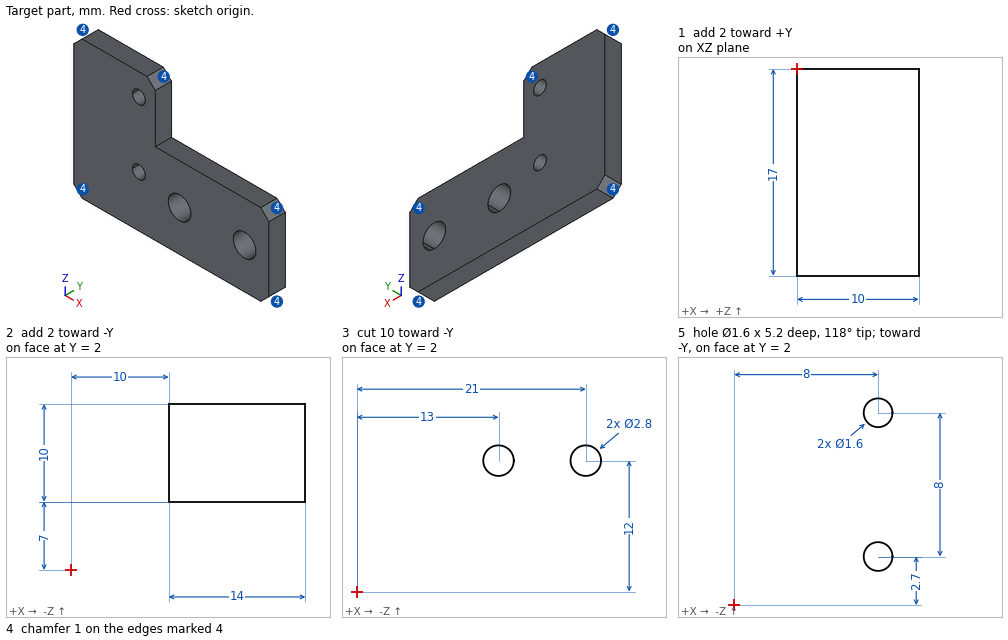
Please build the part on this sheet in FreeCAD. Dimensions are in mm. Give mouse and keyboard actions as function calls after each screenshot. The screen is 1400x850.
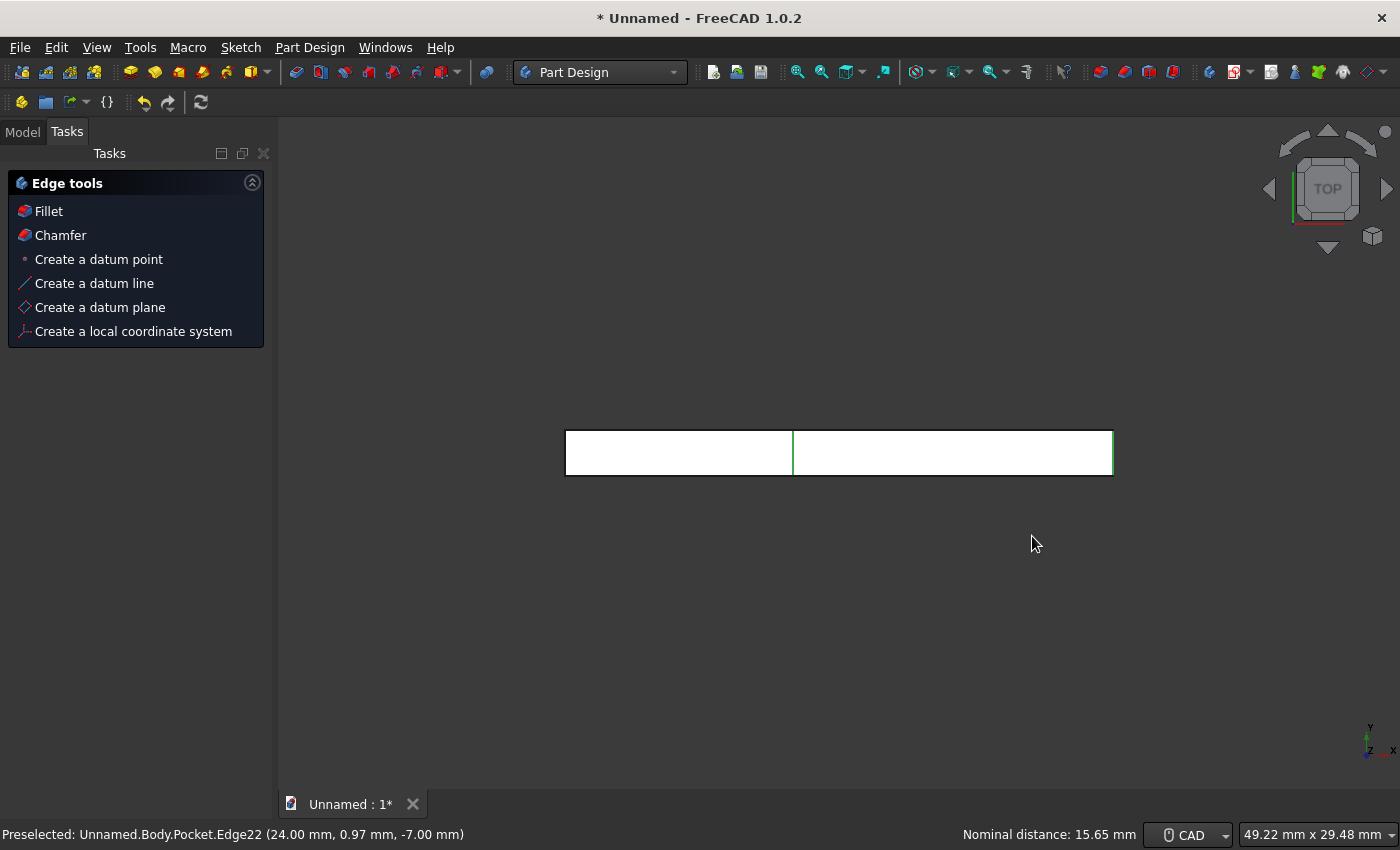
click(565, 452, ctrl)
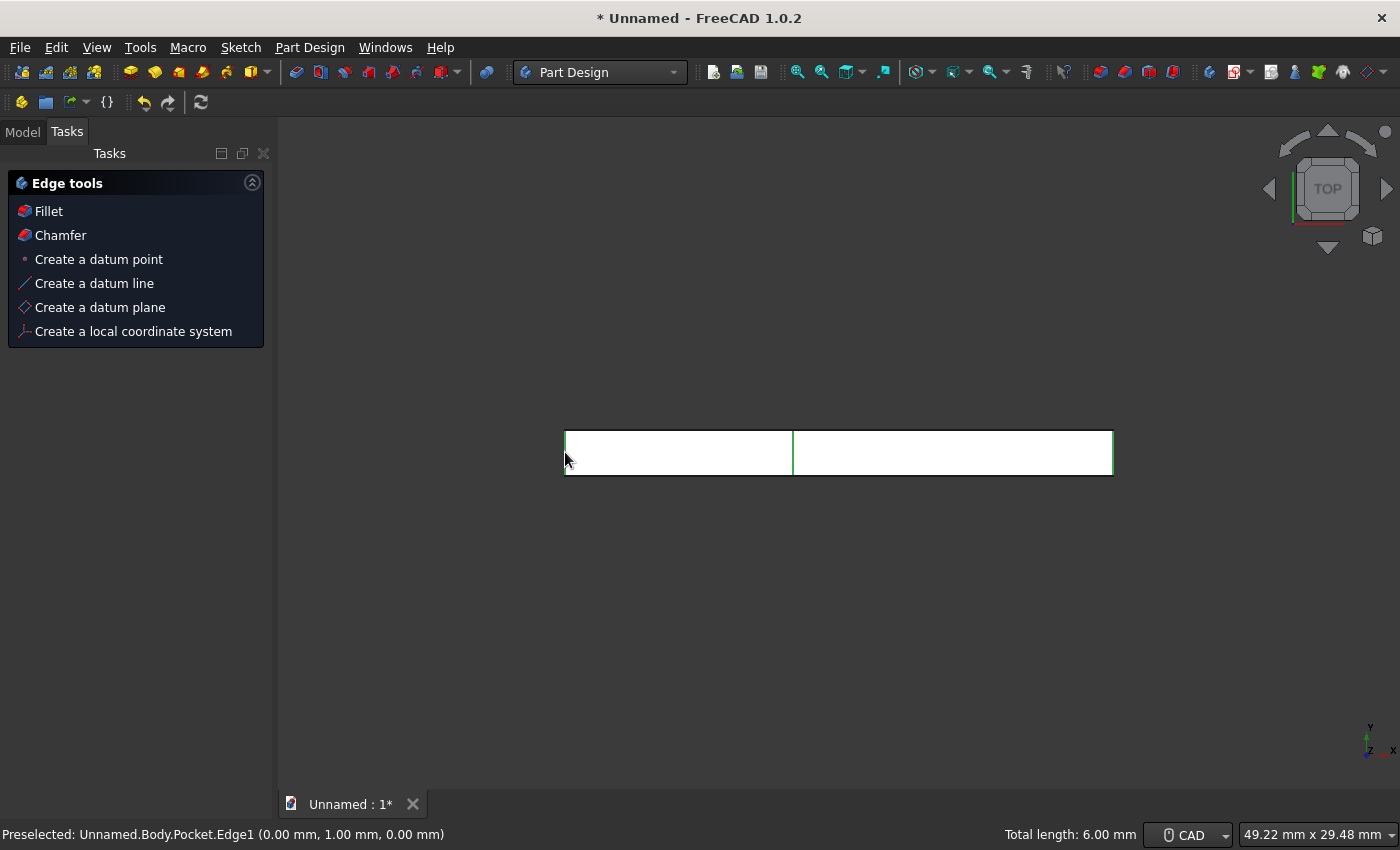
key(1)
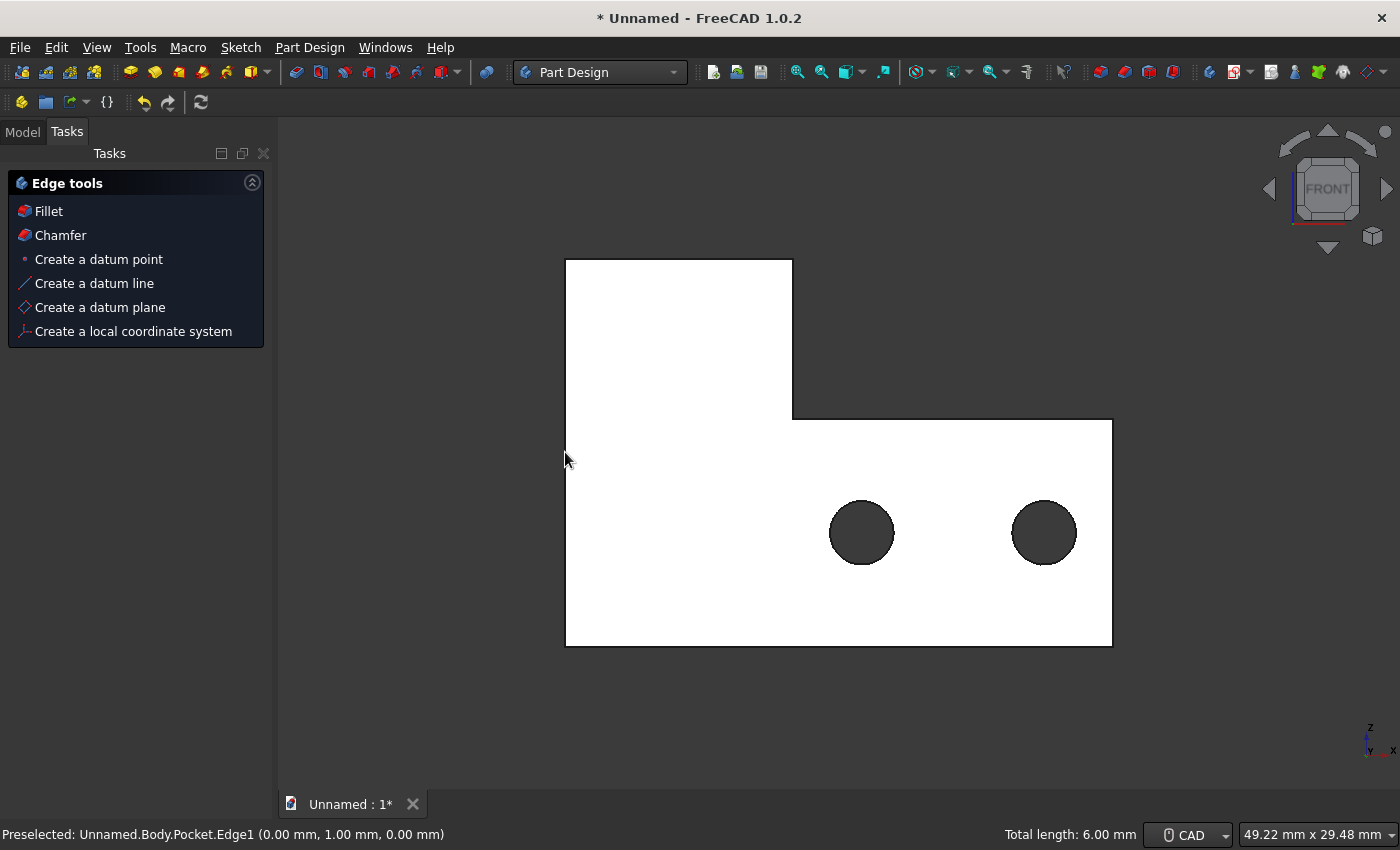
key(3)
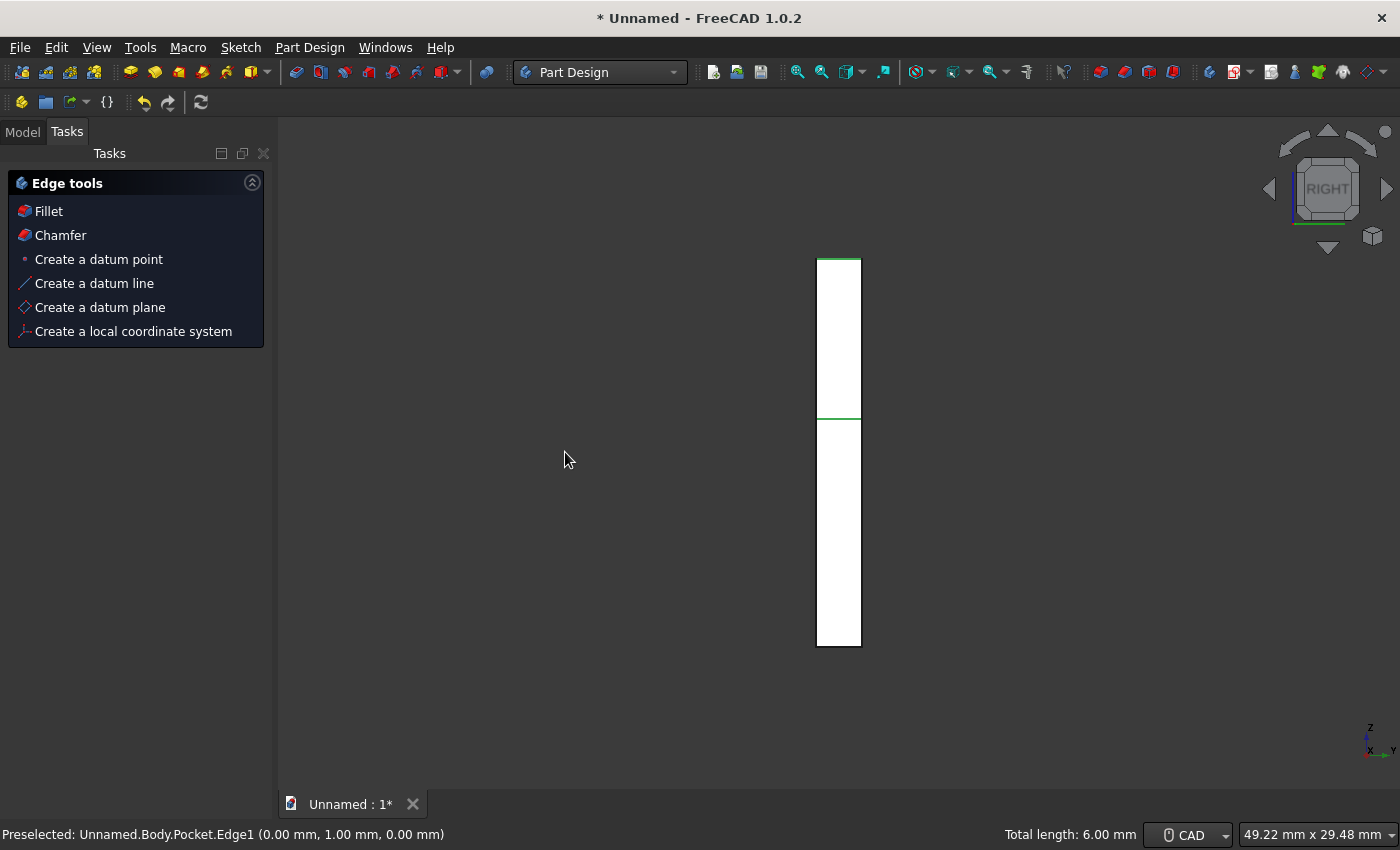
click(839, 646, ctrl)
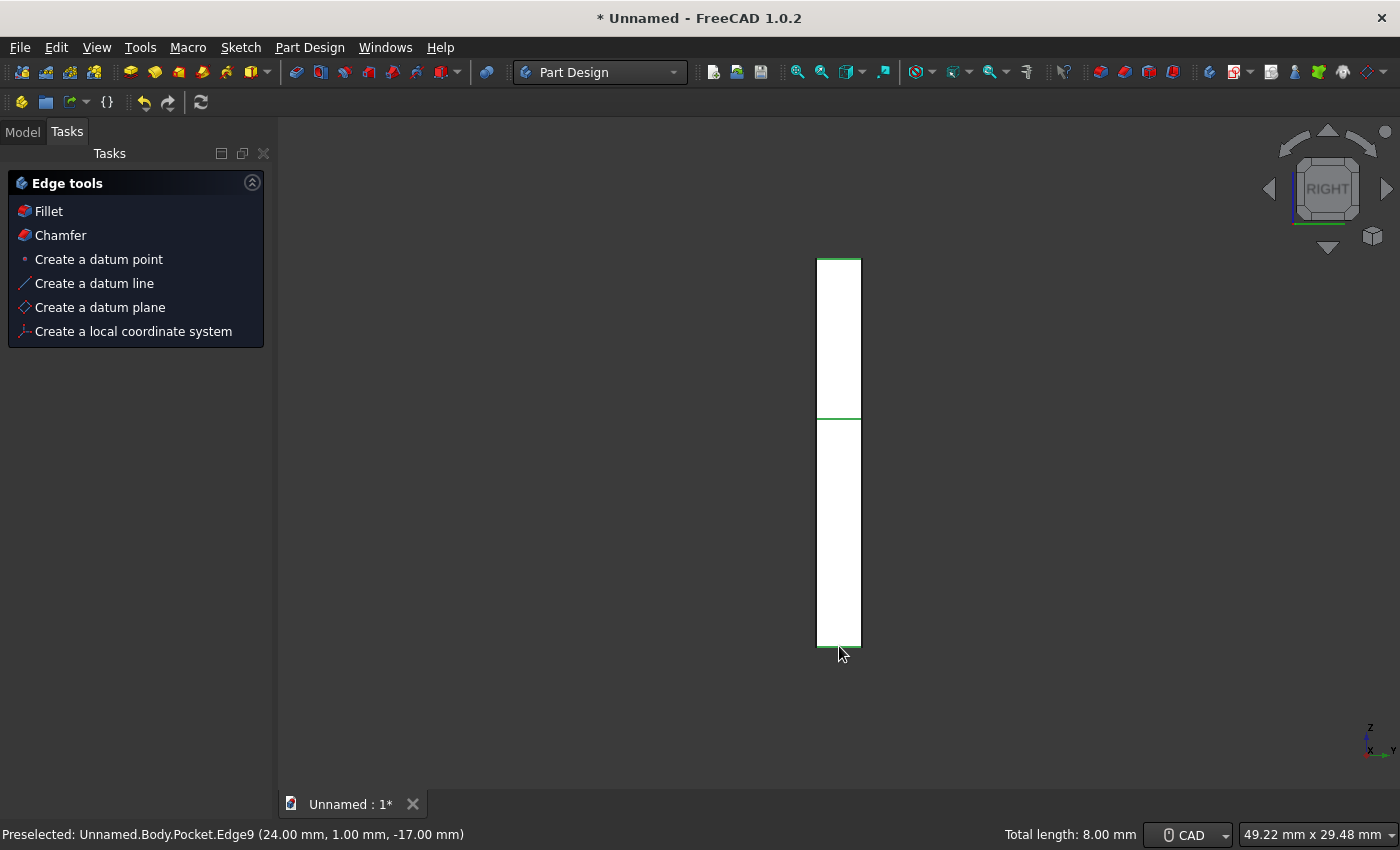
key(5)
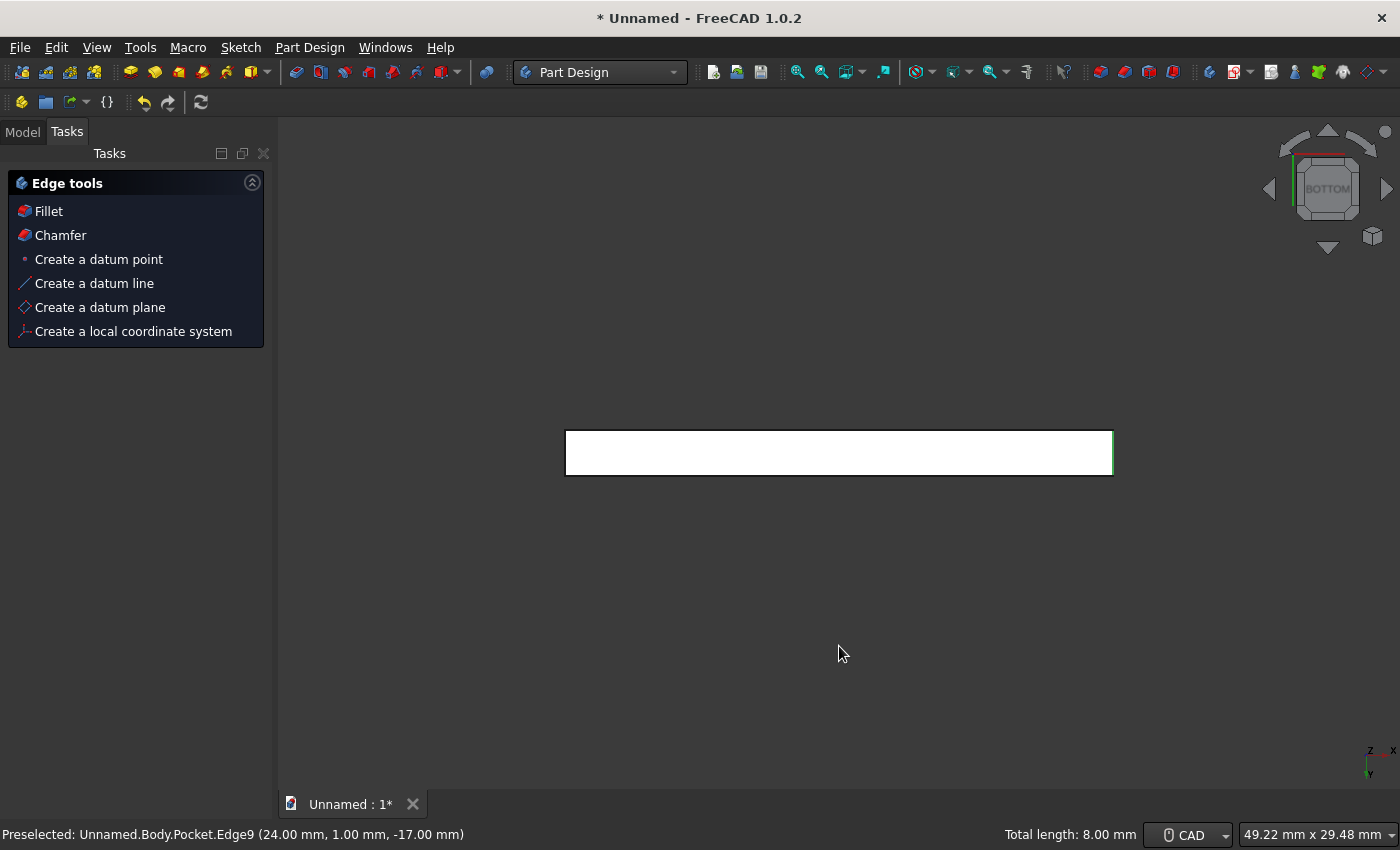
click(565, 452, ctrl)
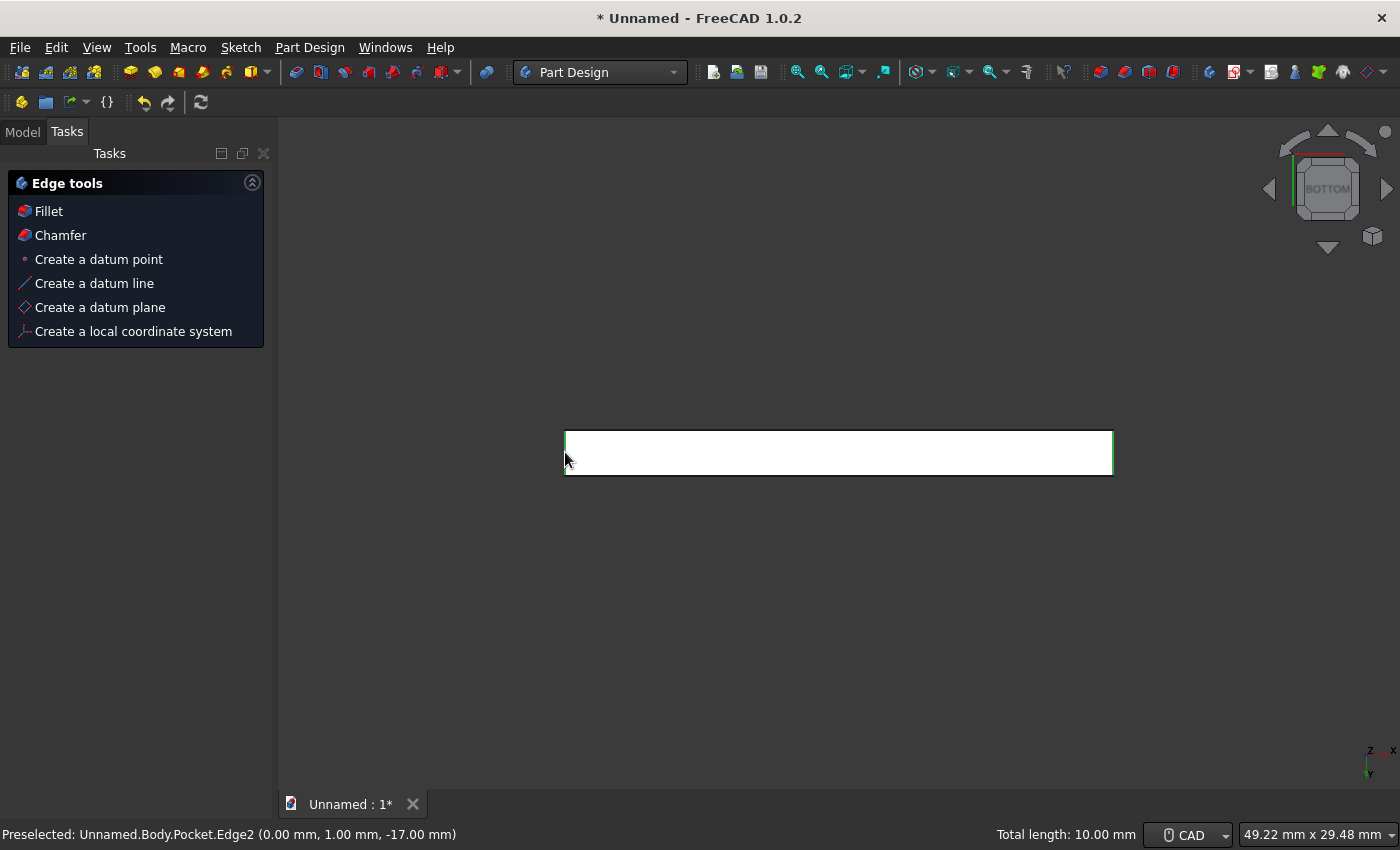
click(1126, 72)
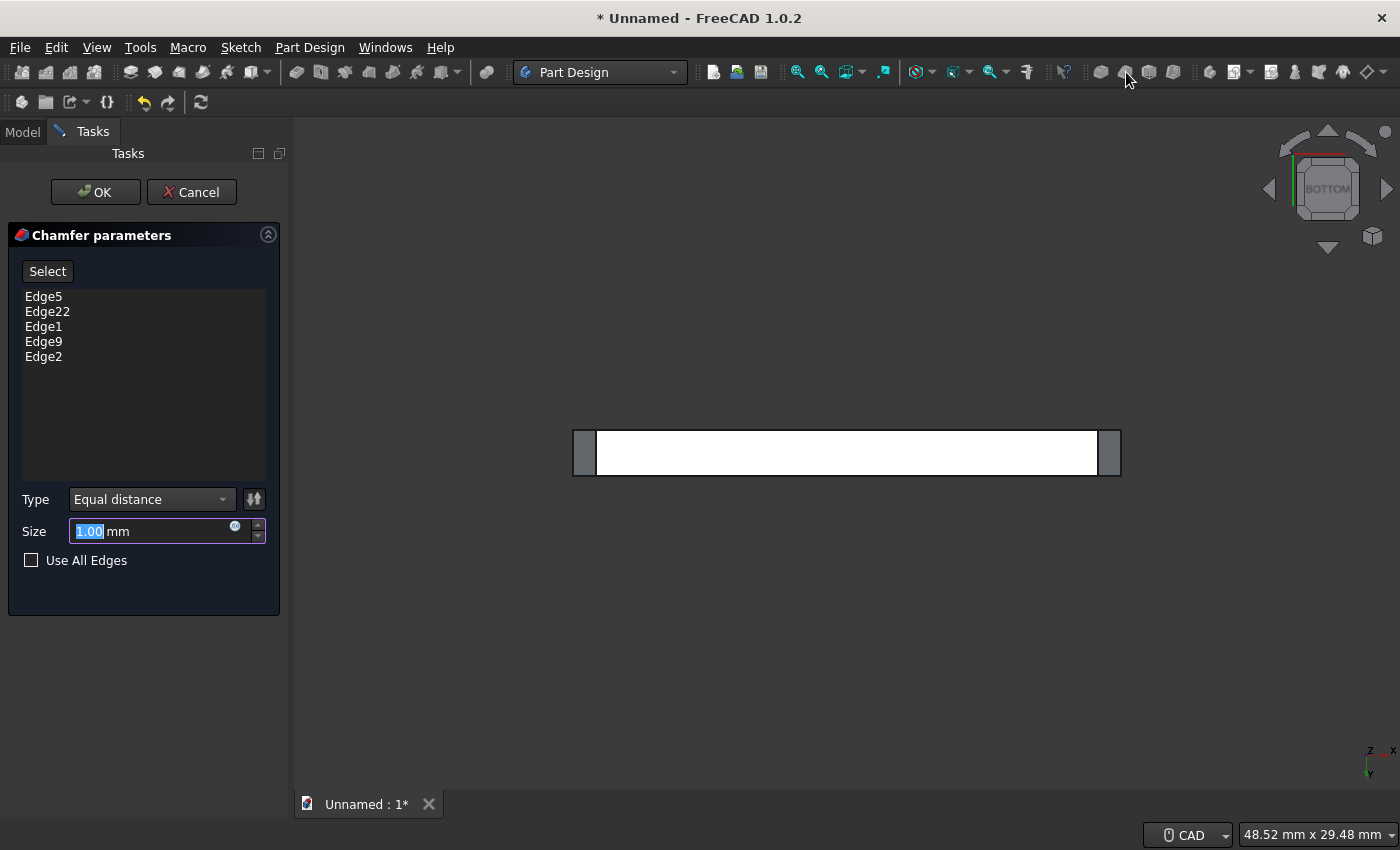
text(1)
key(Tab)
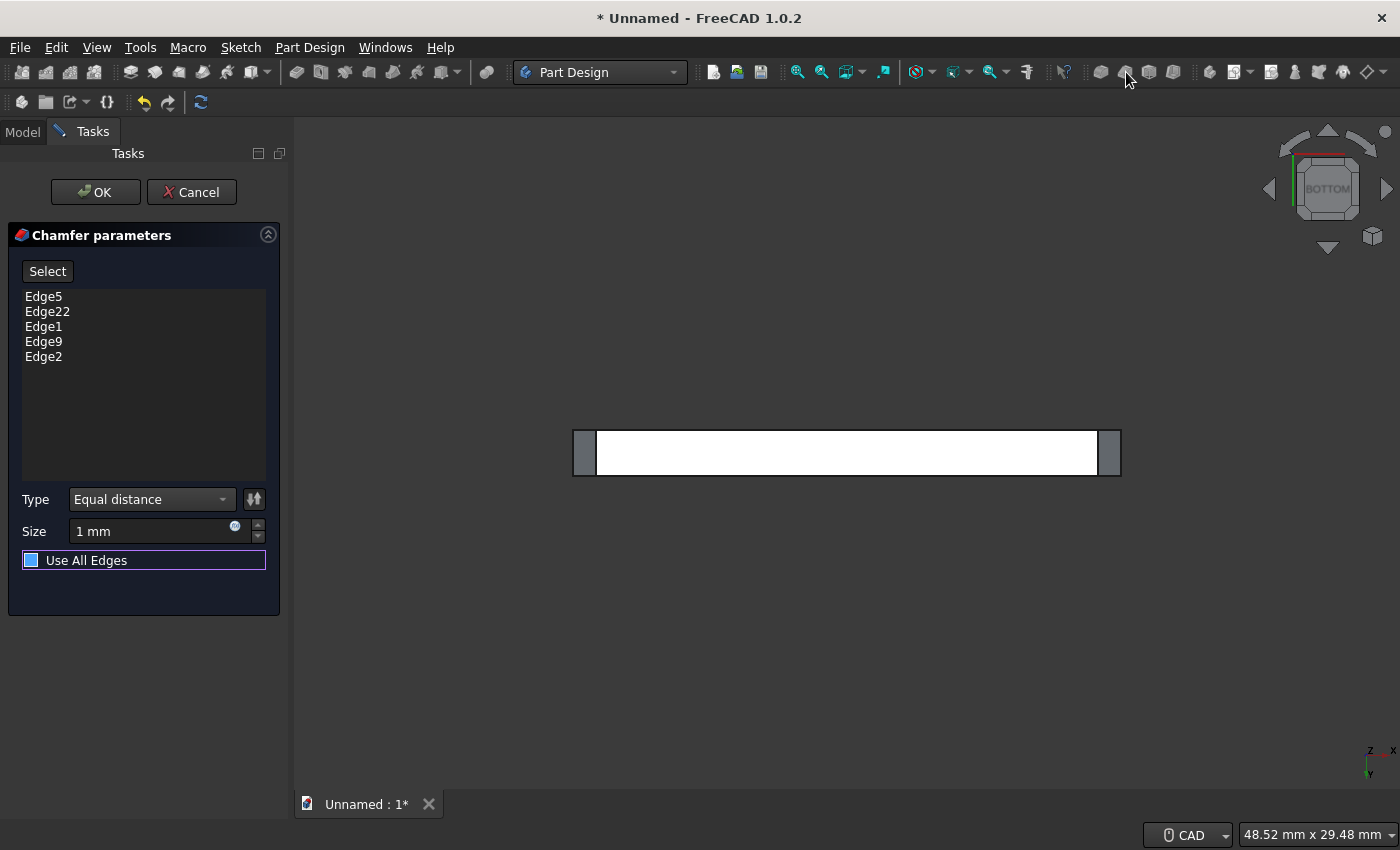
click(96, 192)